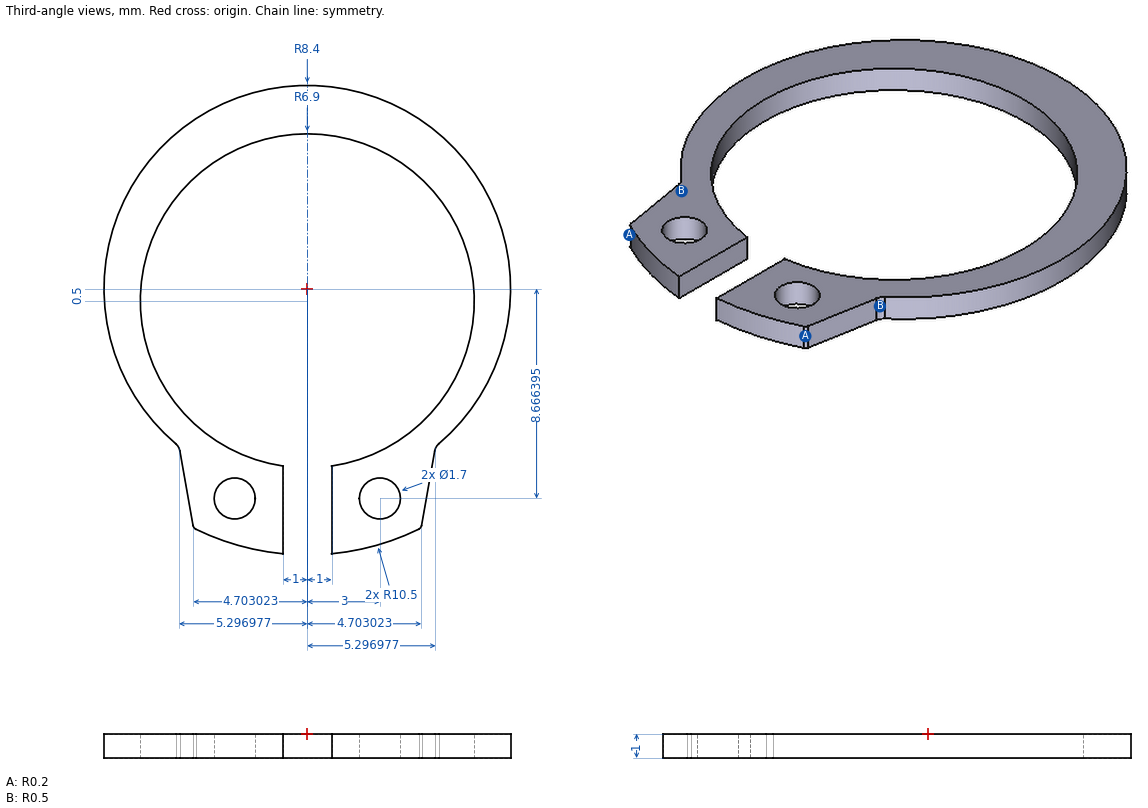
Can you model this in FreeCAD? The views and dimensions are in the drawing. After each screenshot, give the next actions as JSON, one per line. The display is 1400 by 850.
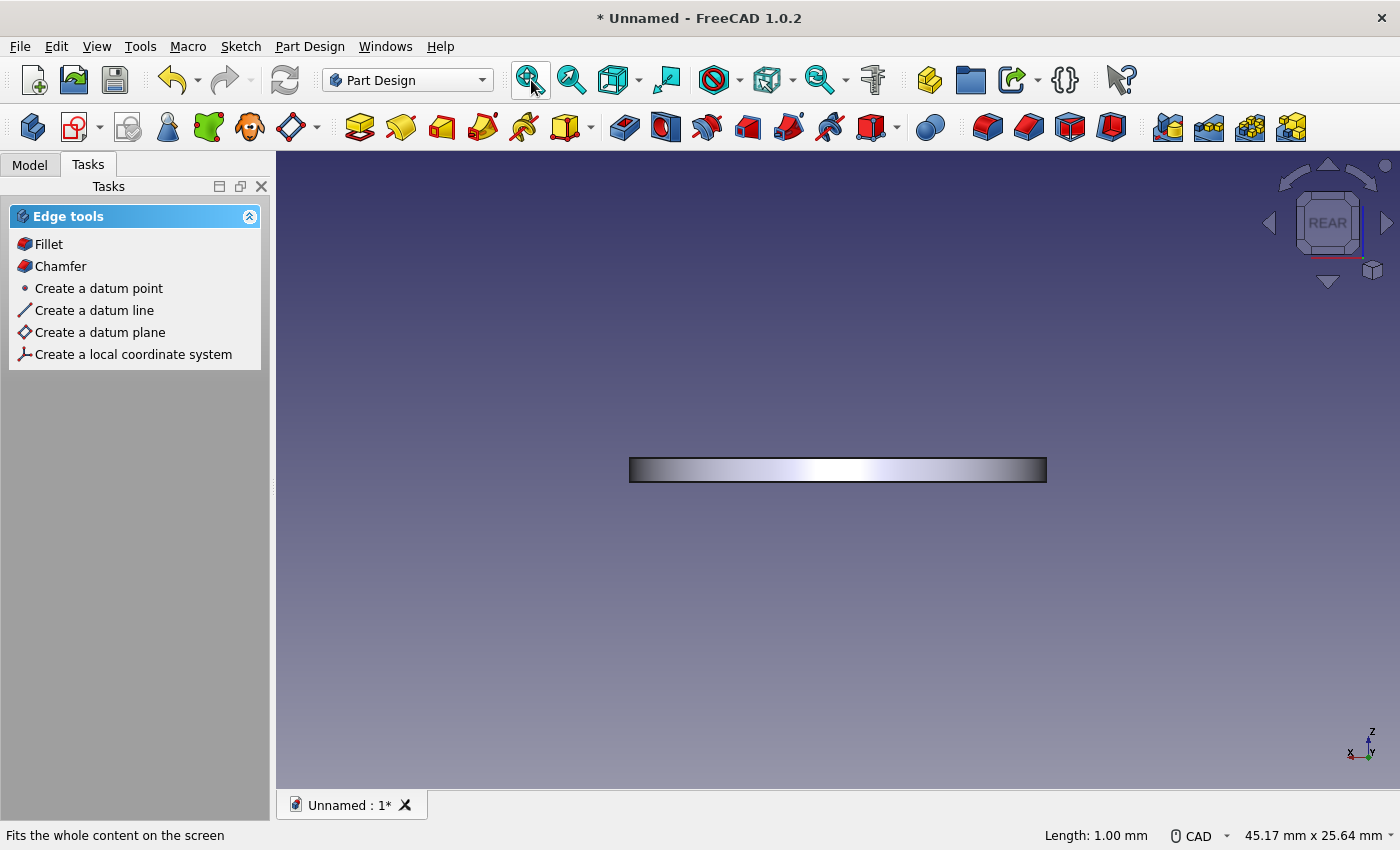
{"action": "key", "text": "6"}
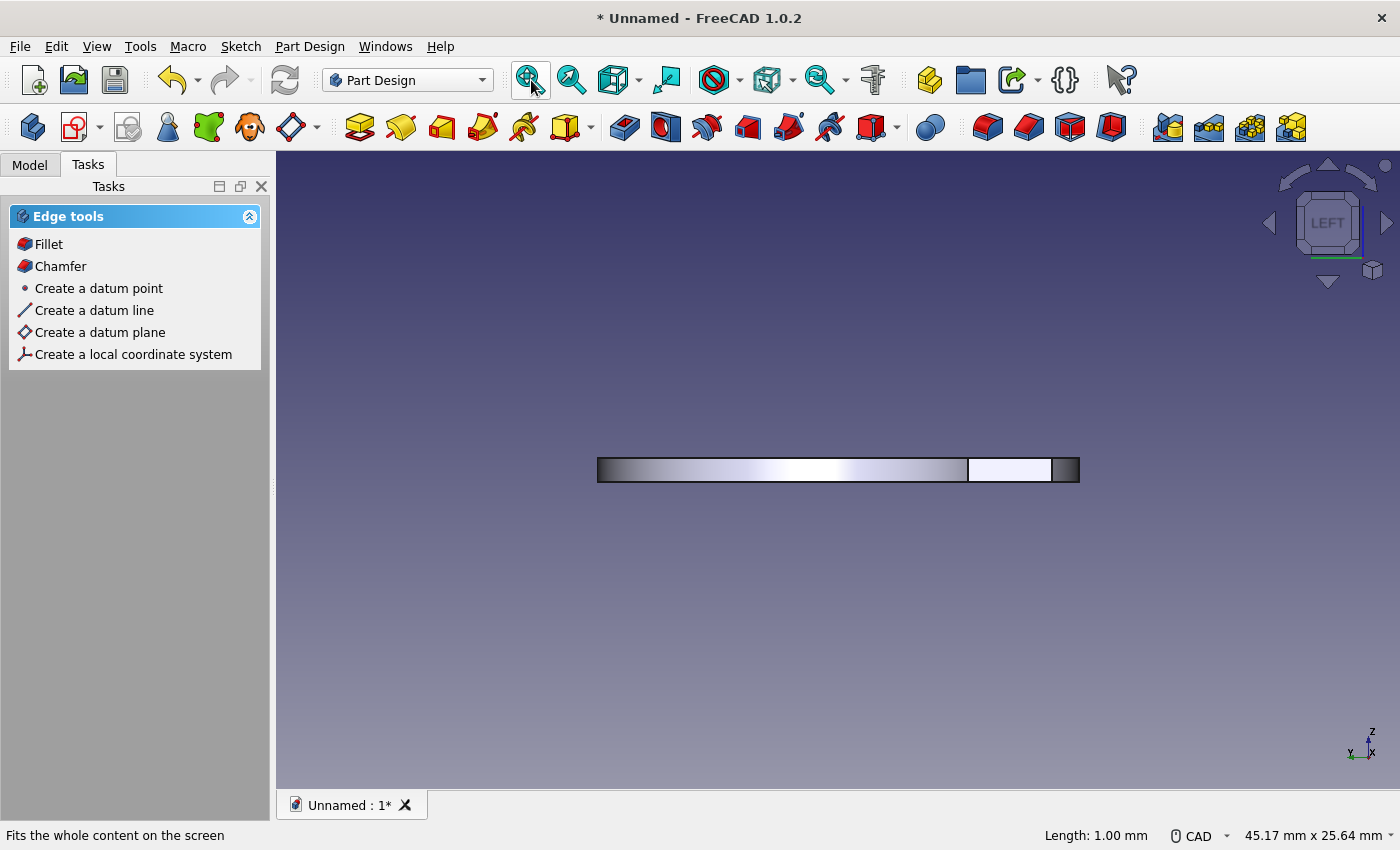
{"action": "left_click", "coordinate": [531, 80]}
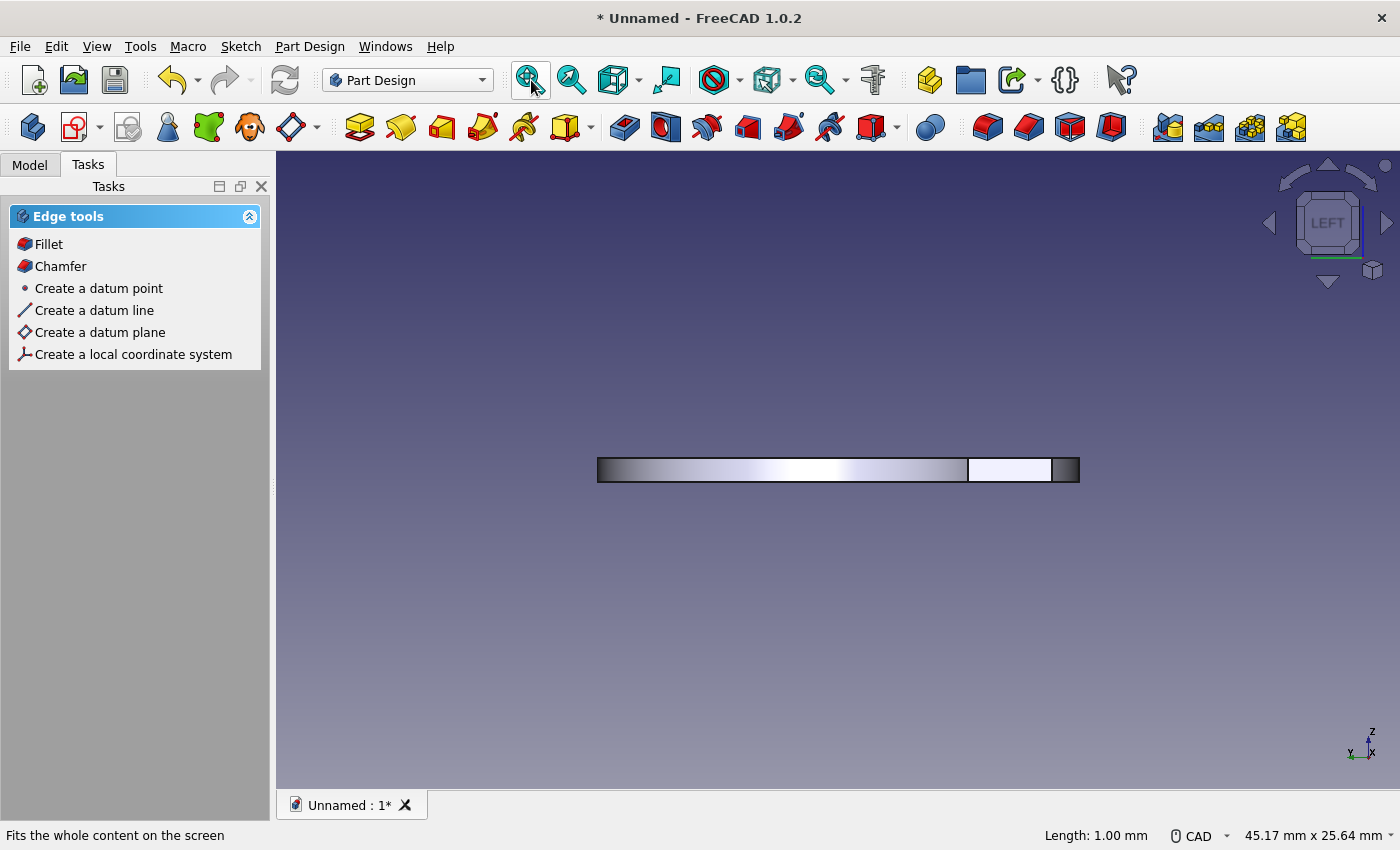
{"action": "key", "text": "v 3"}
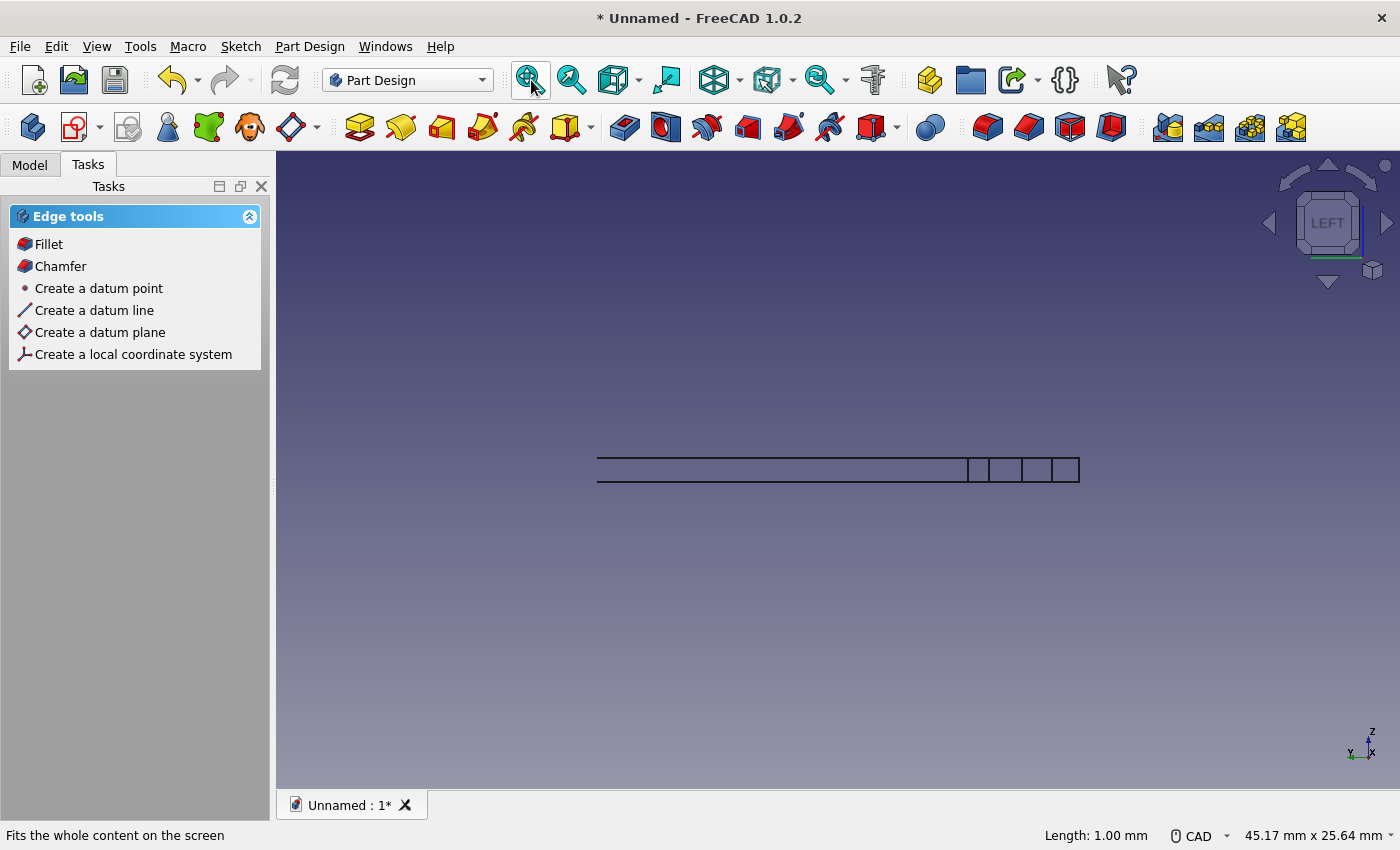
{"action": "key", "text": "0"}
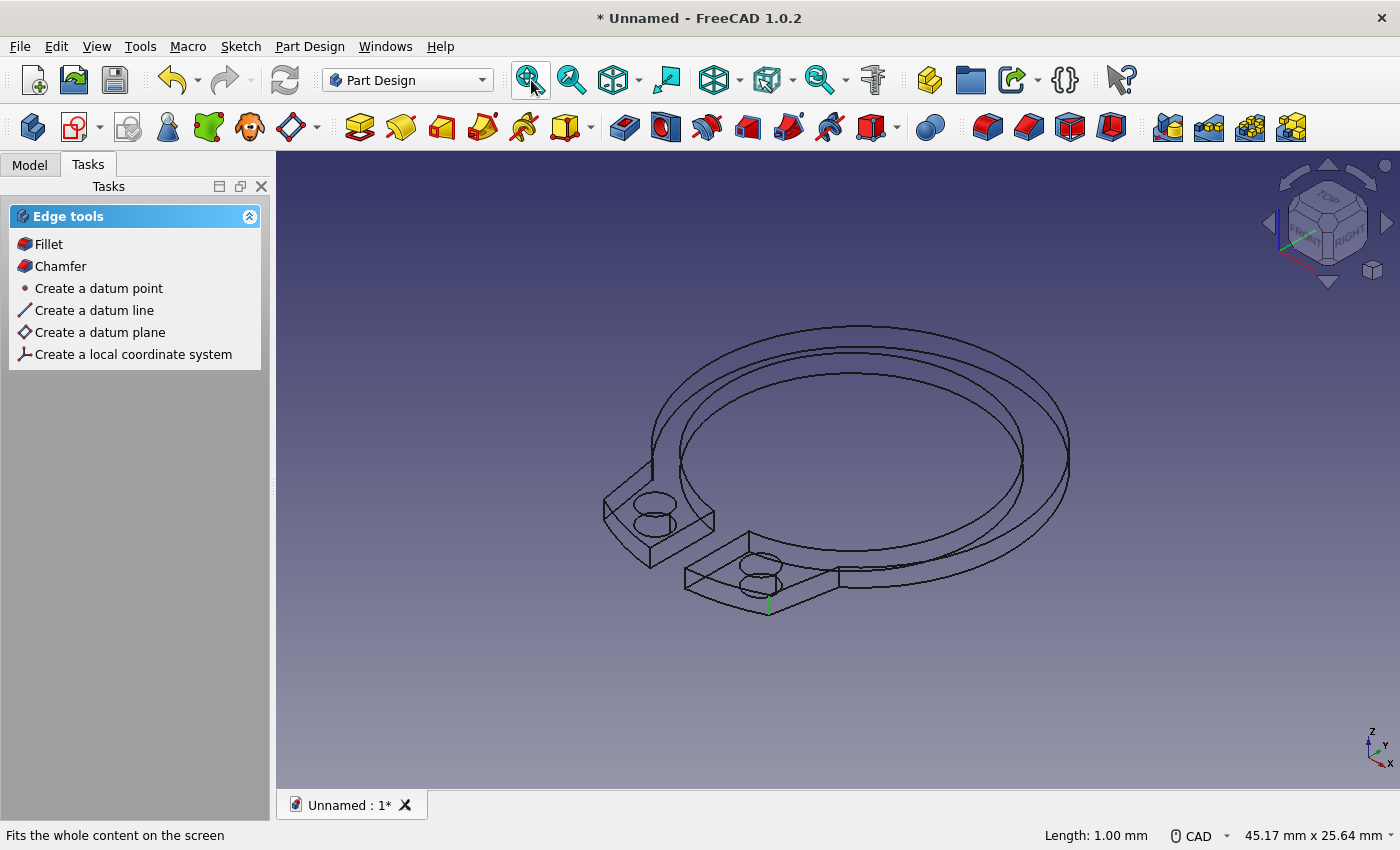
{"action": "left_click", "coordinate": [604, 511], "text": "ctrl"}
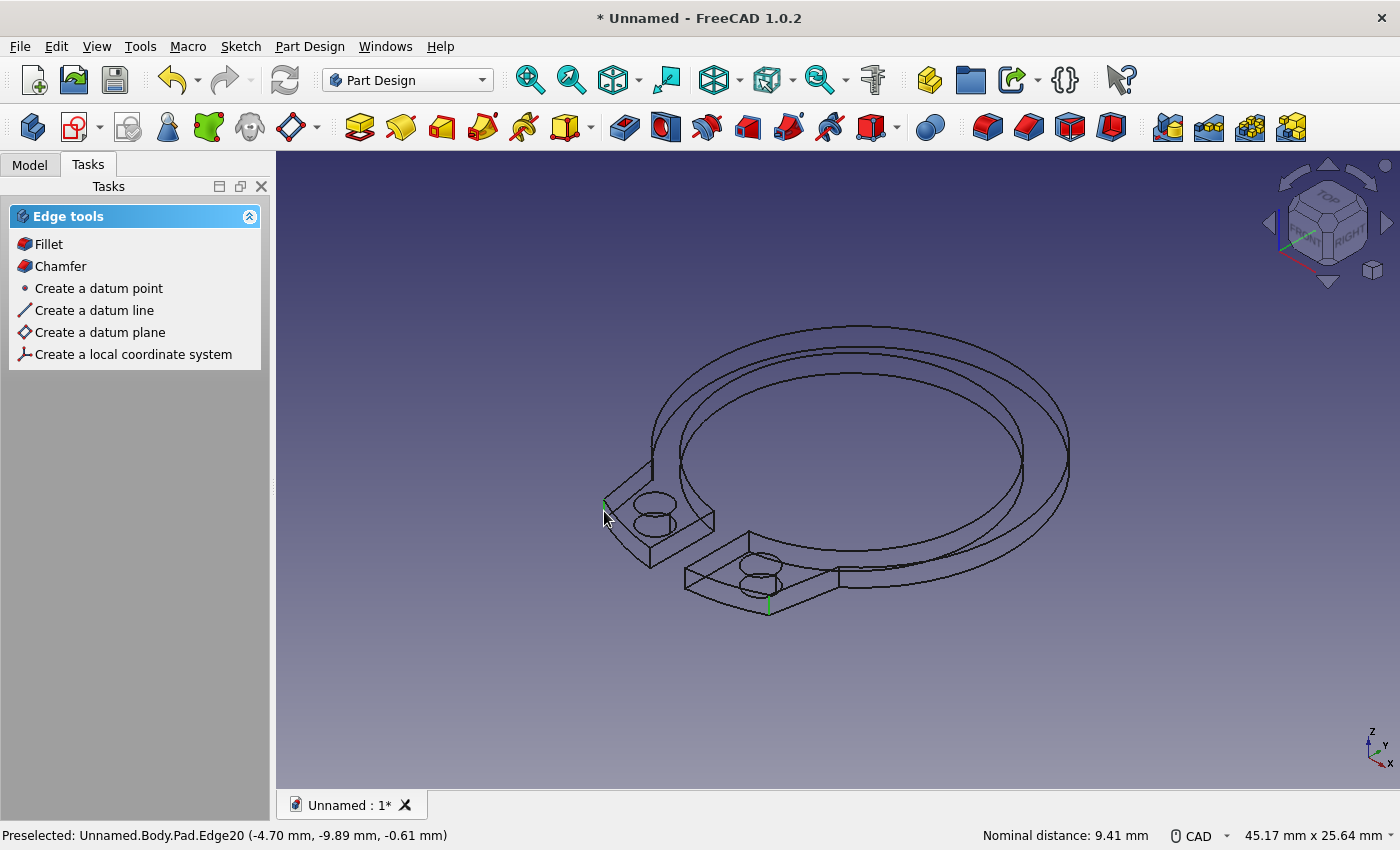
{"action": "key", "text": "v 1"}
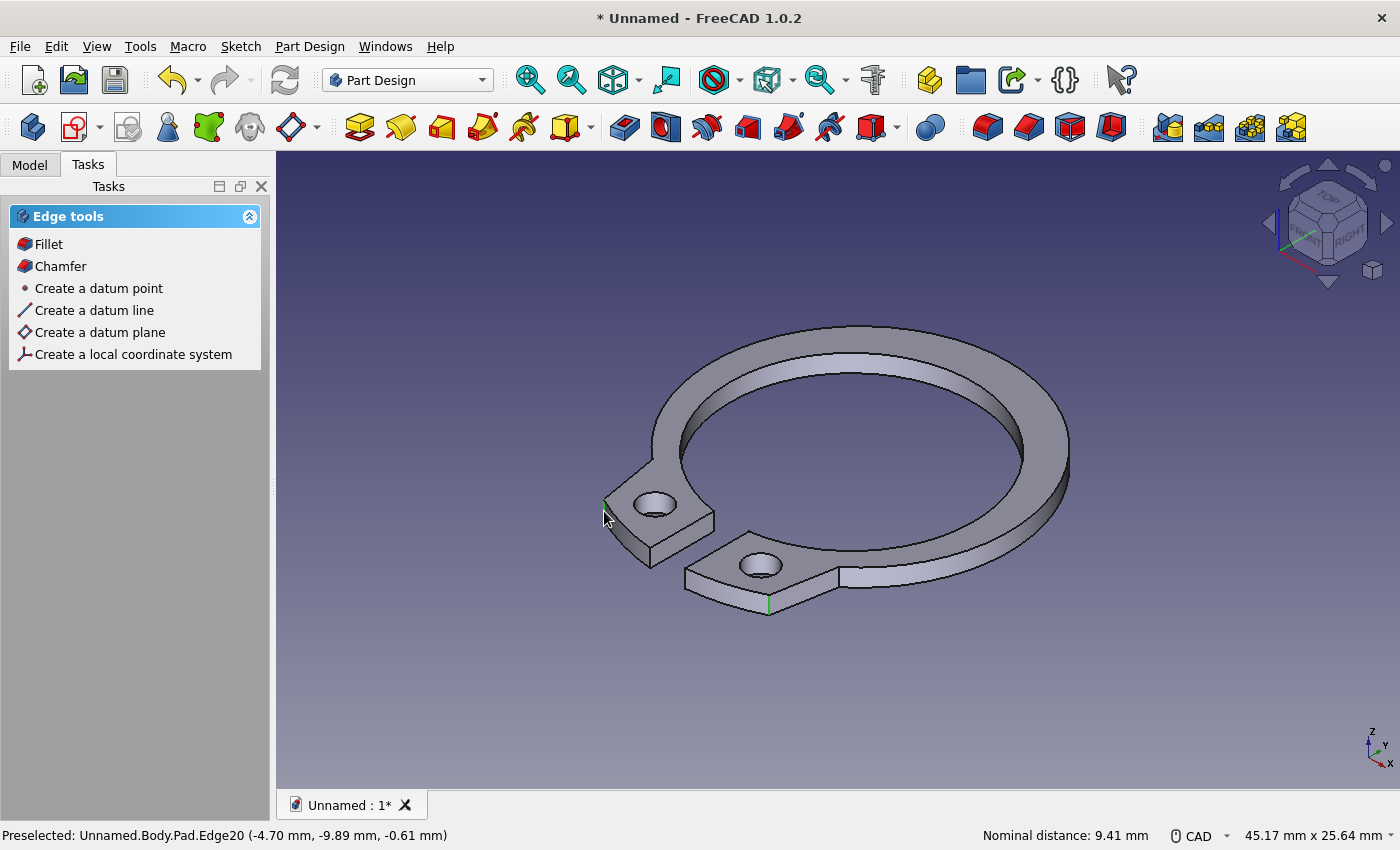
{"action": "left_click", "coordinate": [988, 128]}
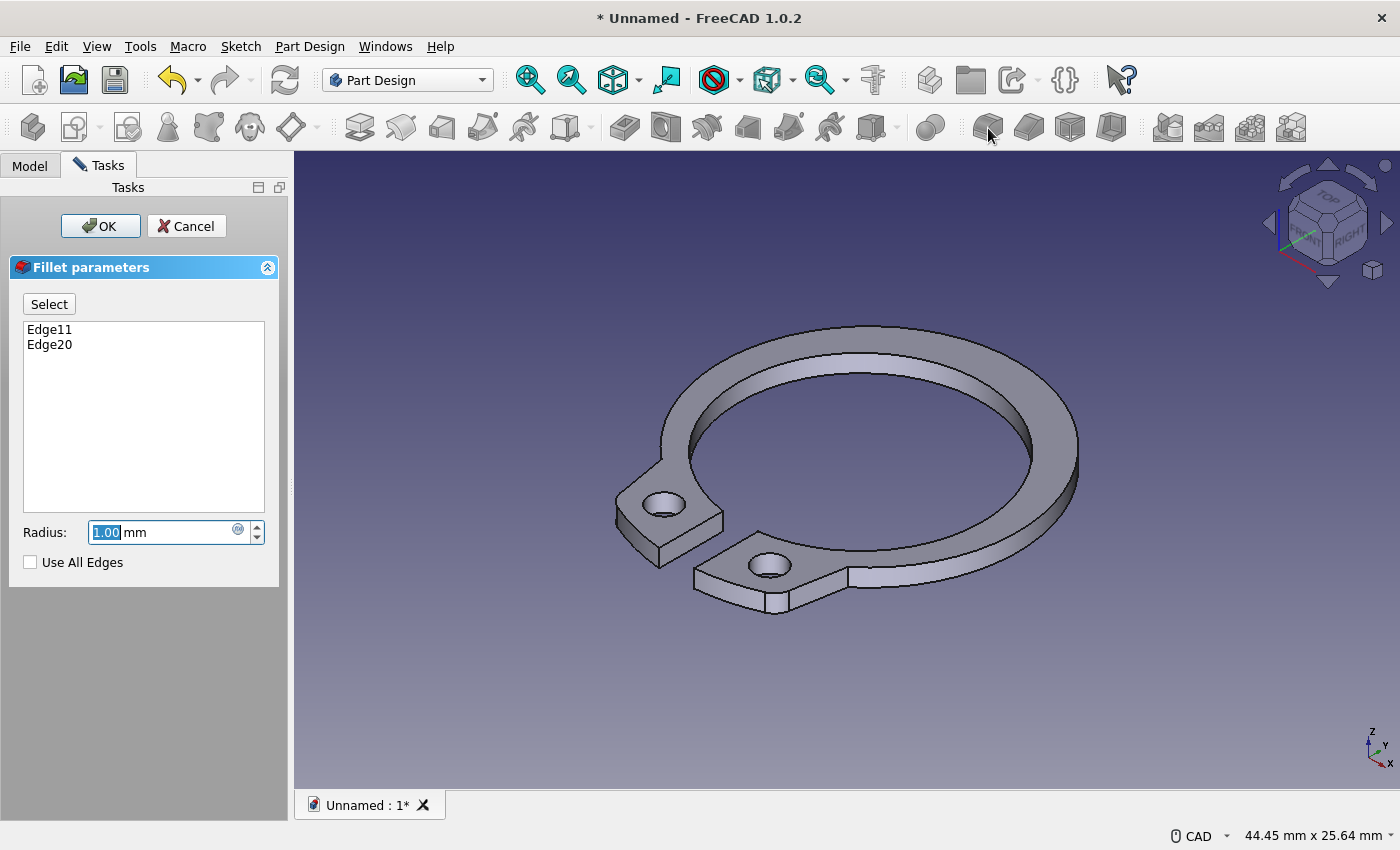
{"action": "type", "text": "0.2"}
{"action": "key", "text": "Tab"}